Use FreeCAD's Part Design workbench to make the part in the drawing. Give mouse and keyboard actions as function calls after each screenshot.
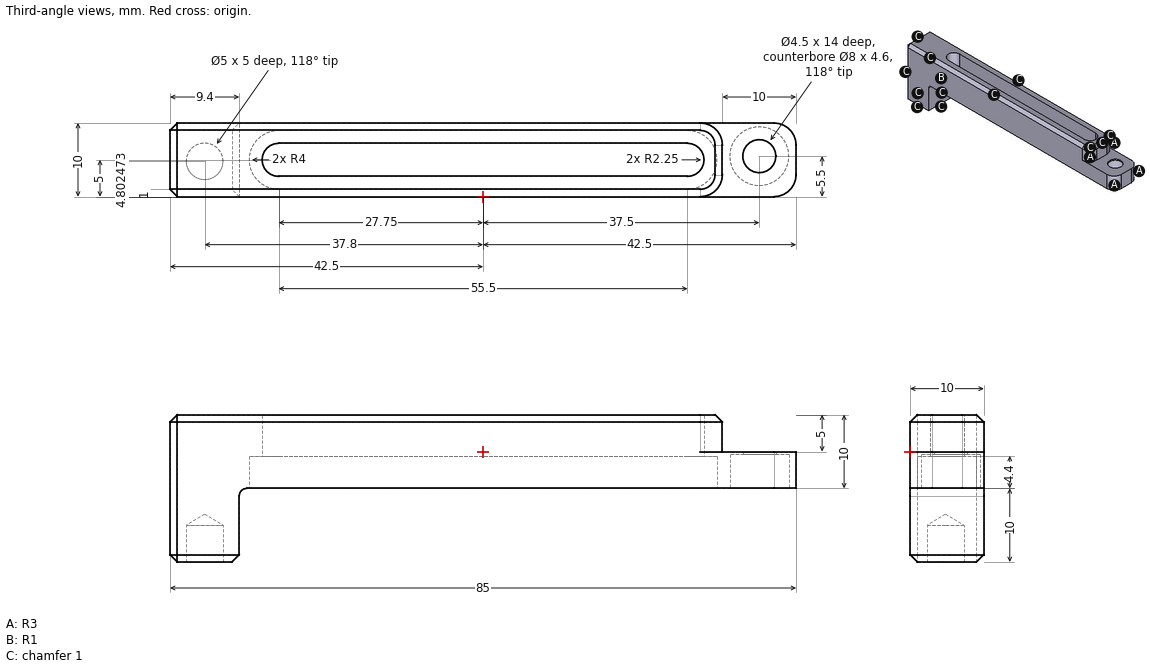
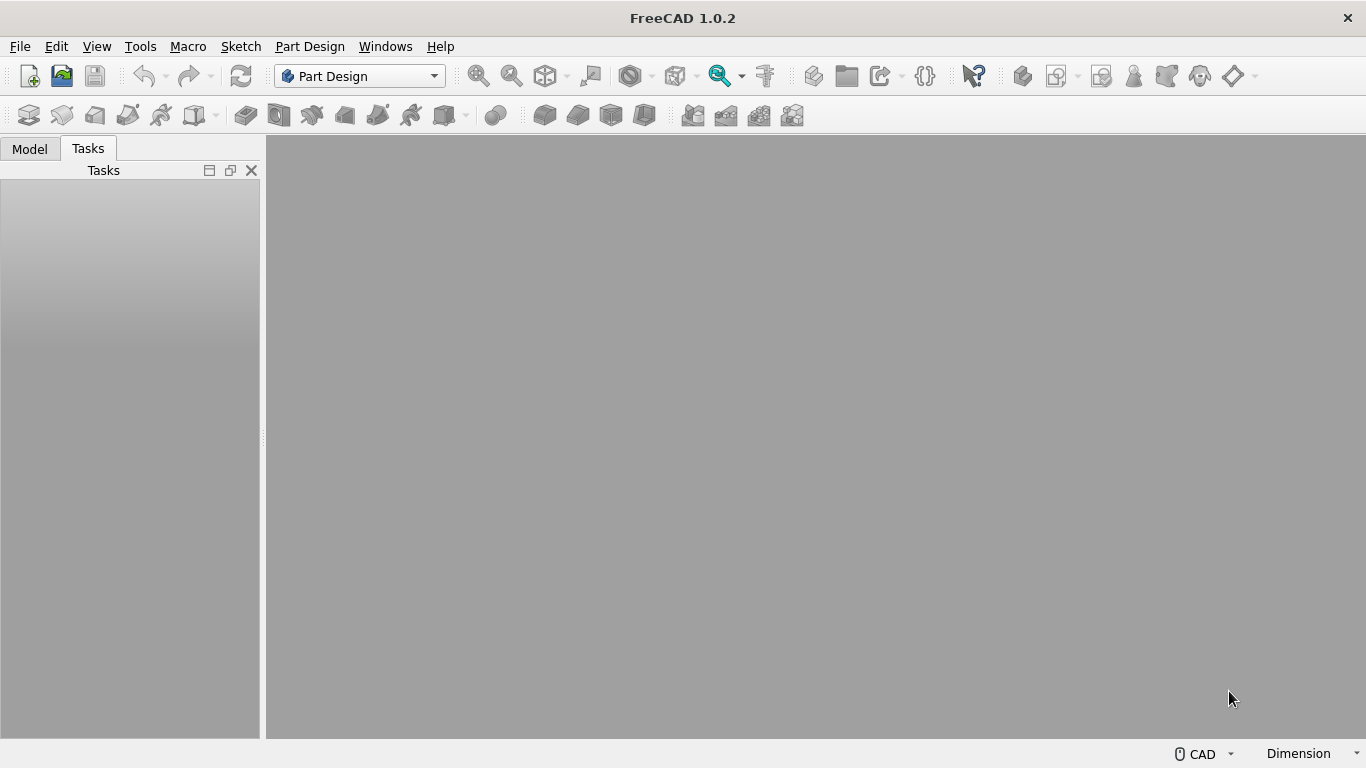
click(29, 76)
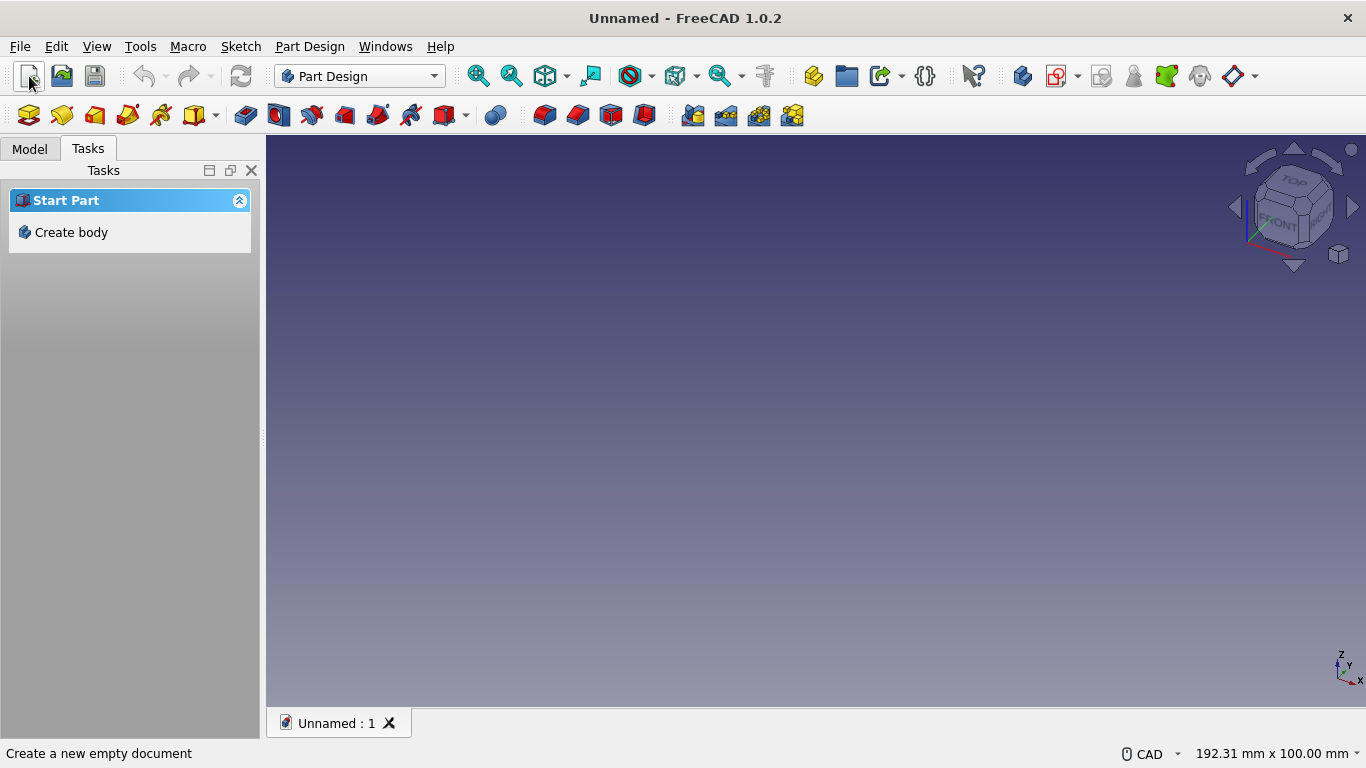
click(1056, 76)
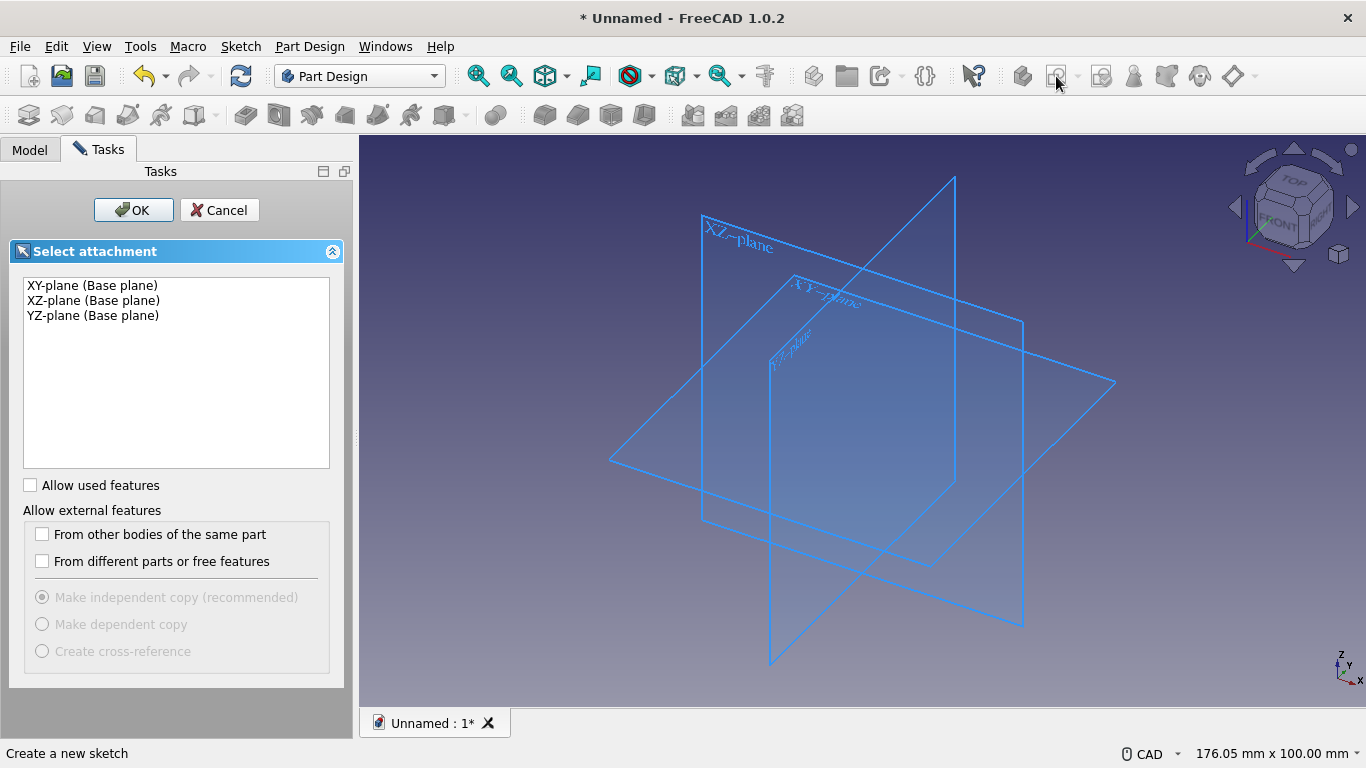
click(84, 300)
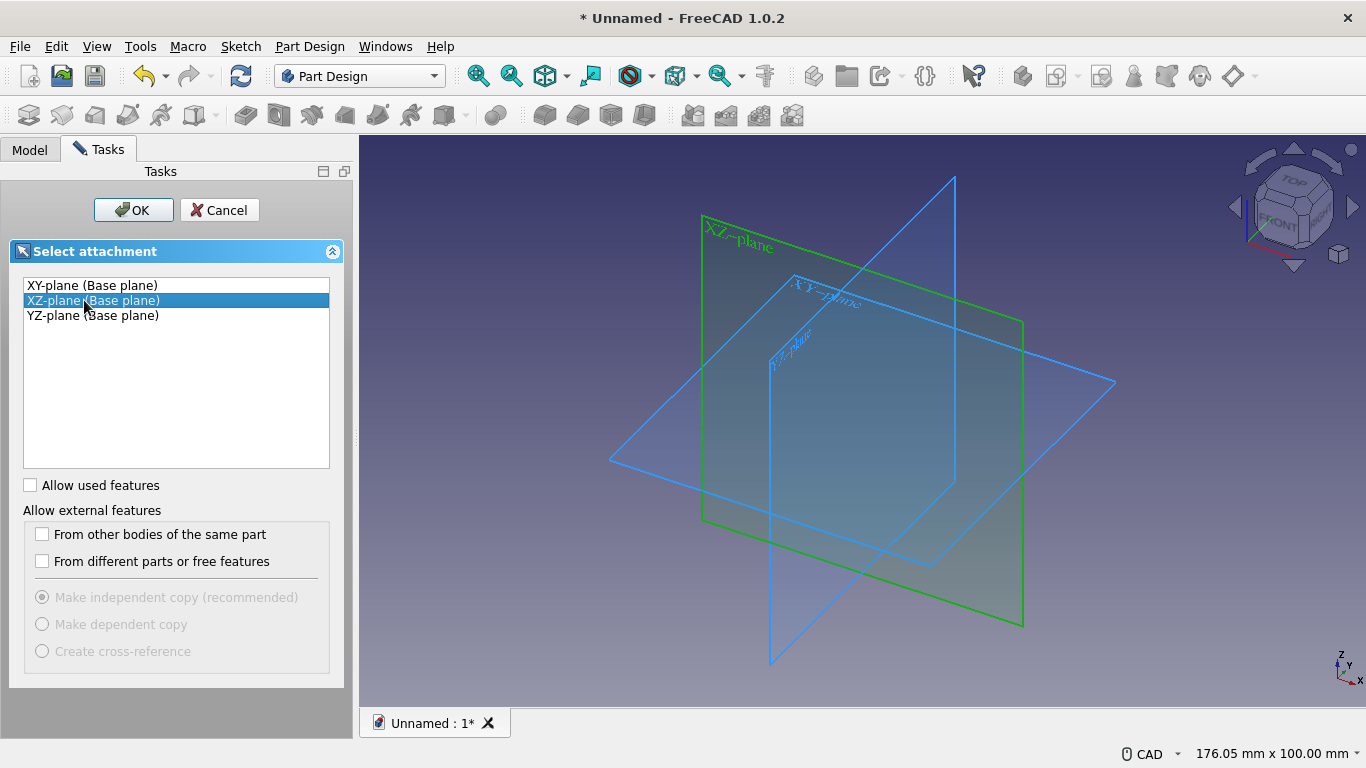
click(134, 210)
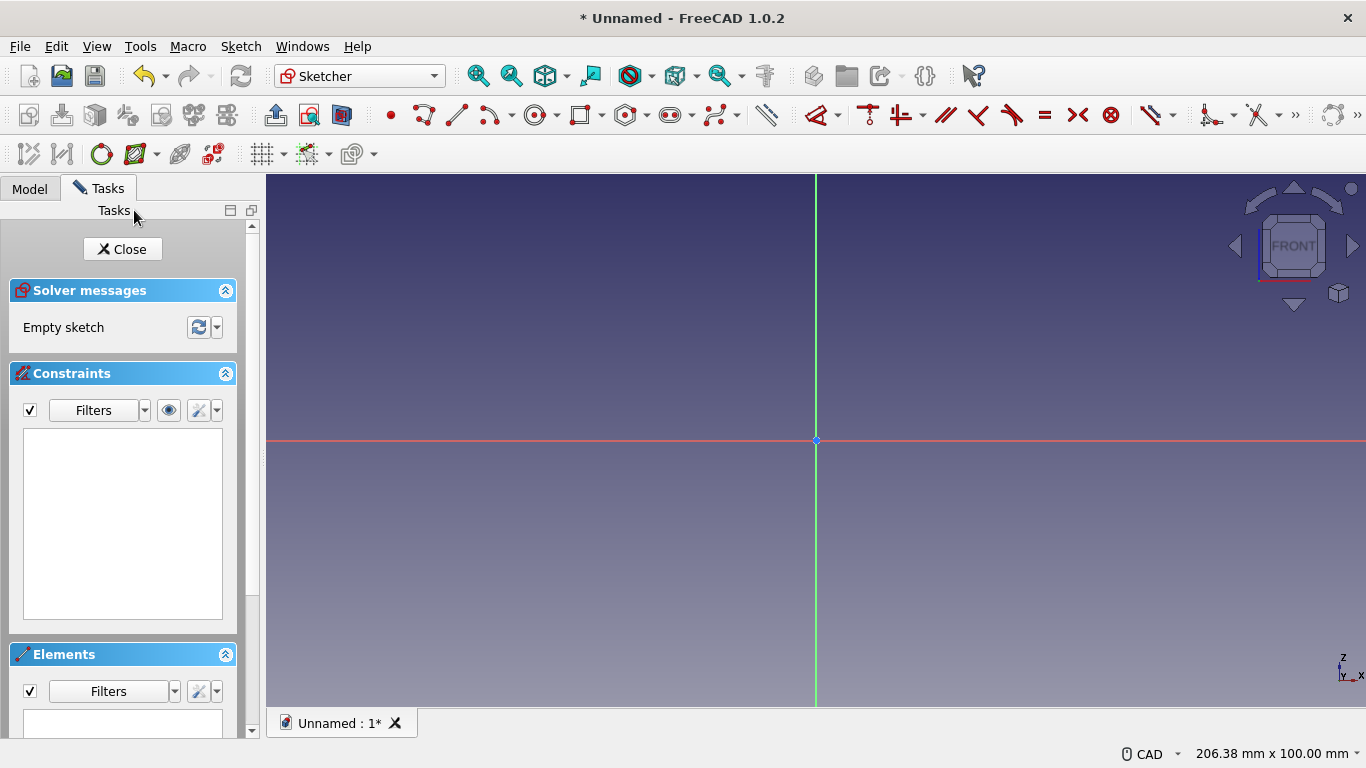
scroll(955, 440, up, 2)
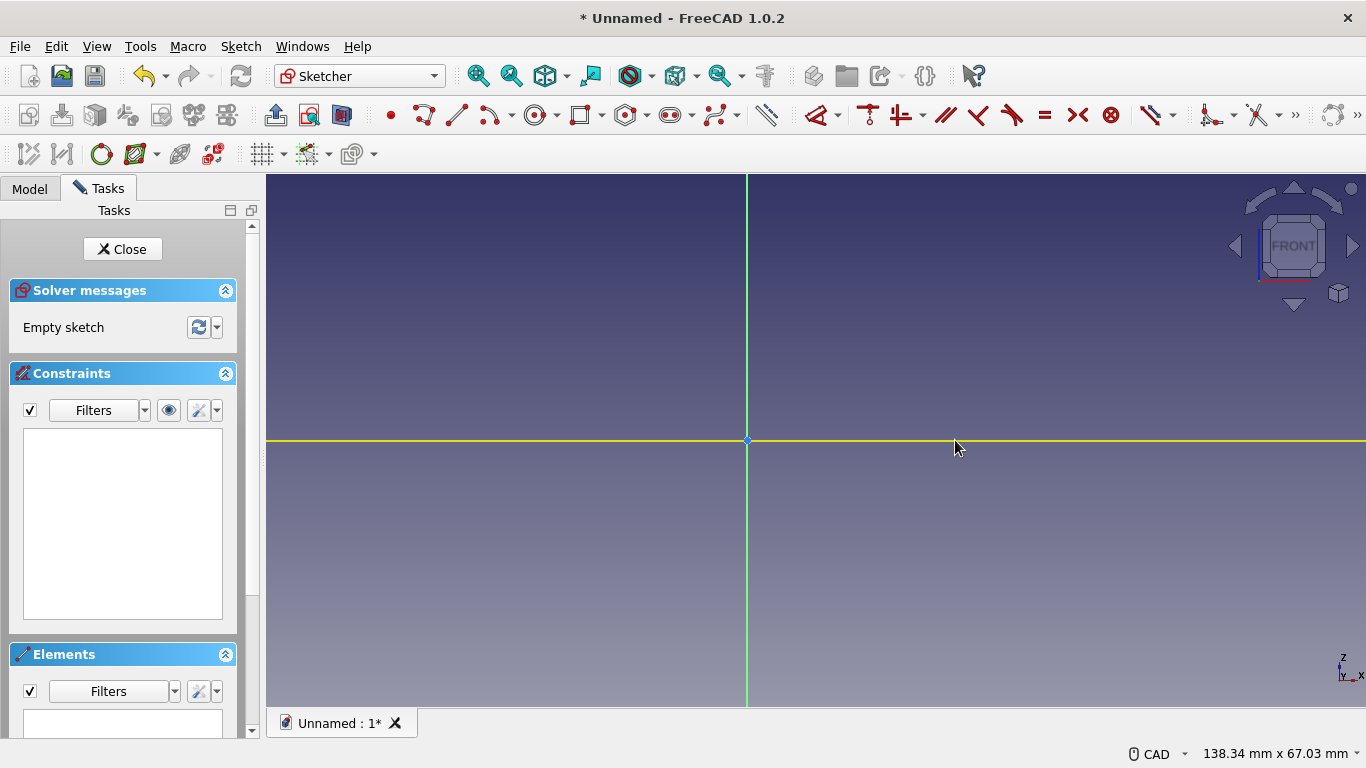
key(g)
key(v)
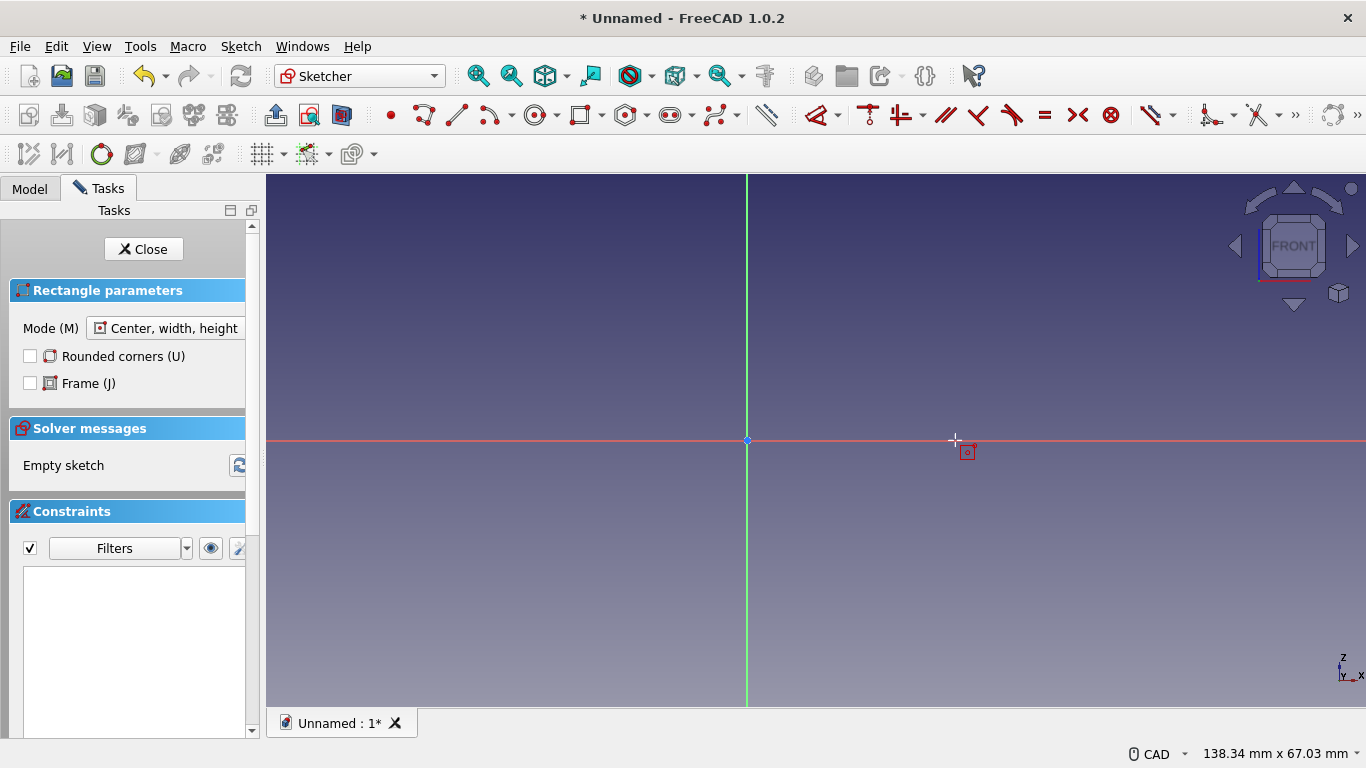
click(747, 440)
click(1085, 401)
key(Escape)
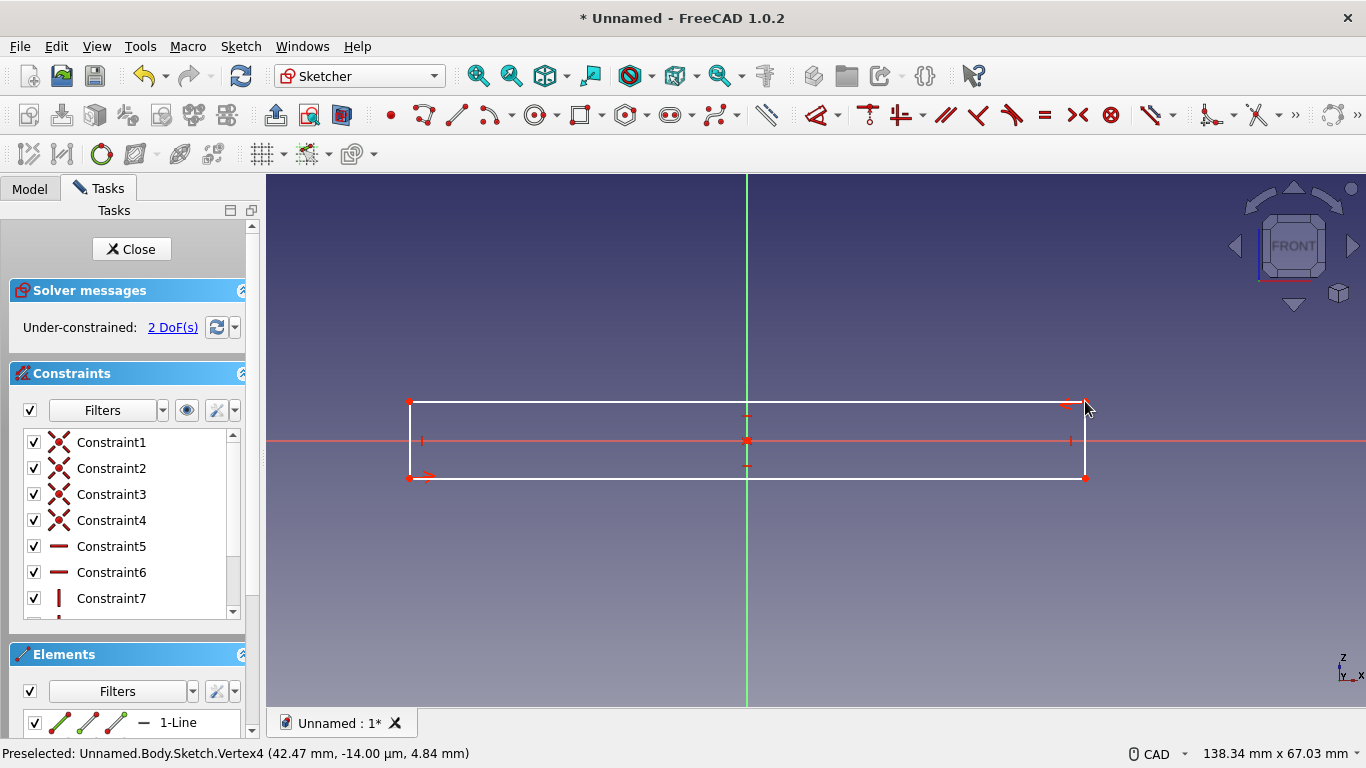
click(816, 116)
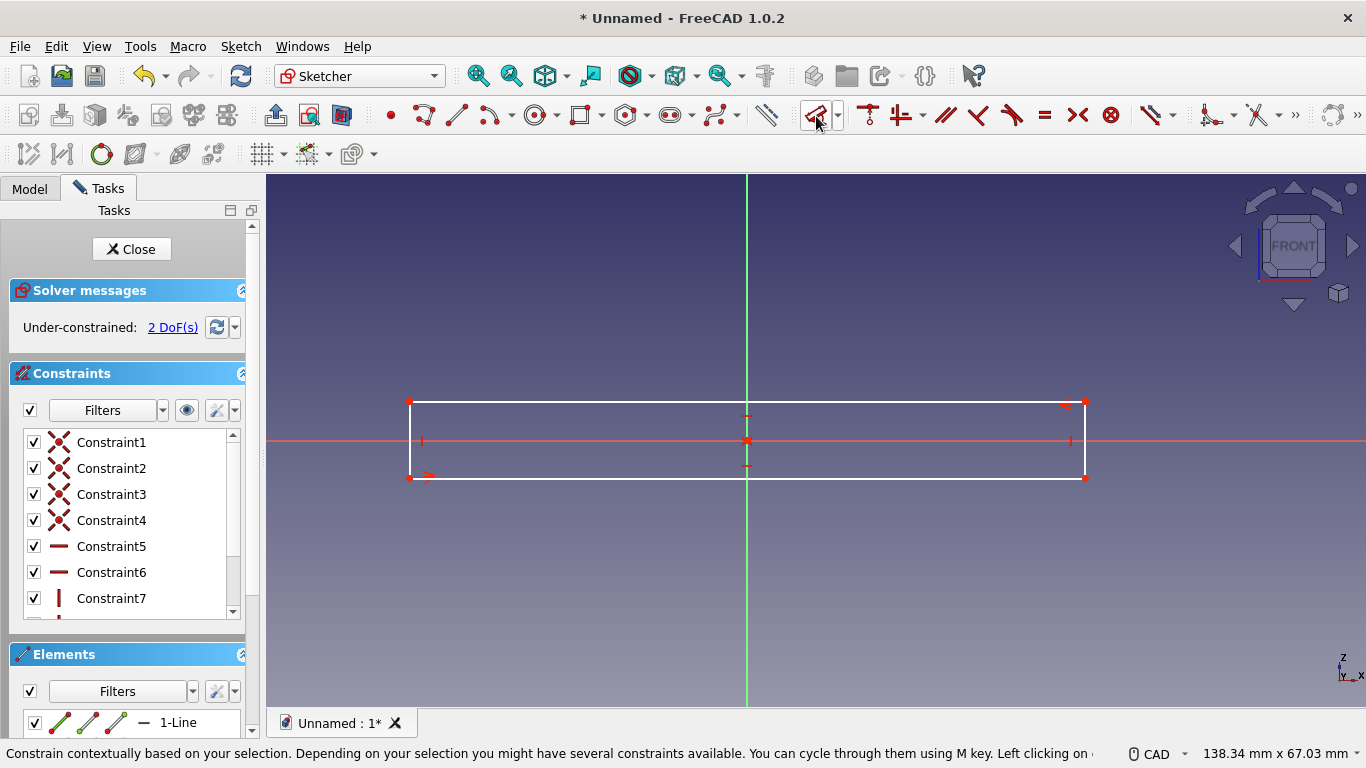
click(612, 479)
click(592, 513)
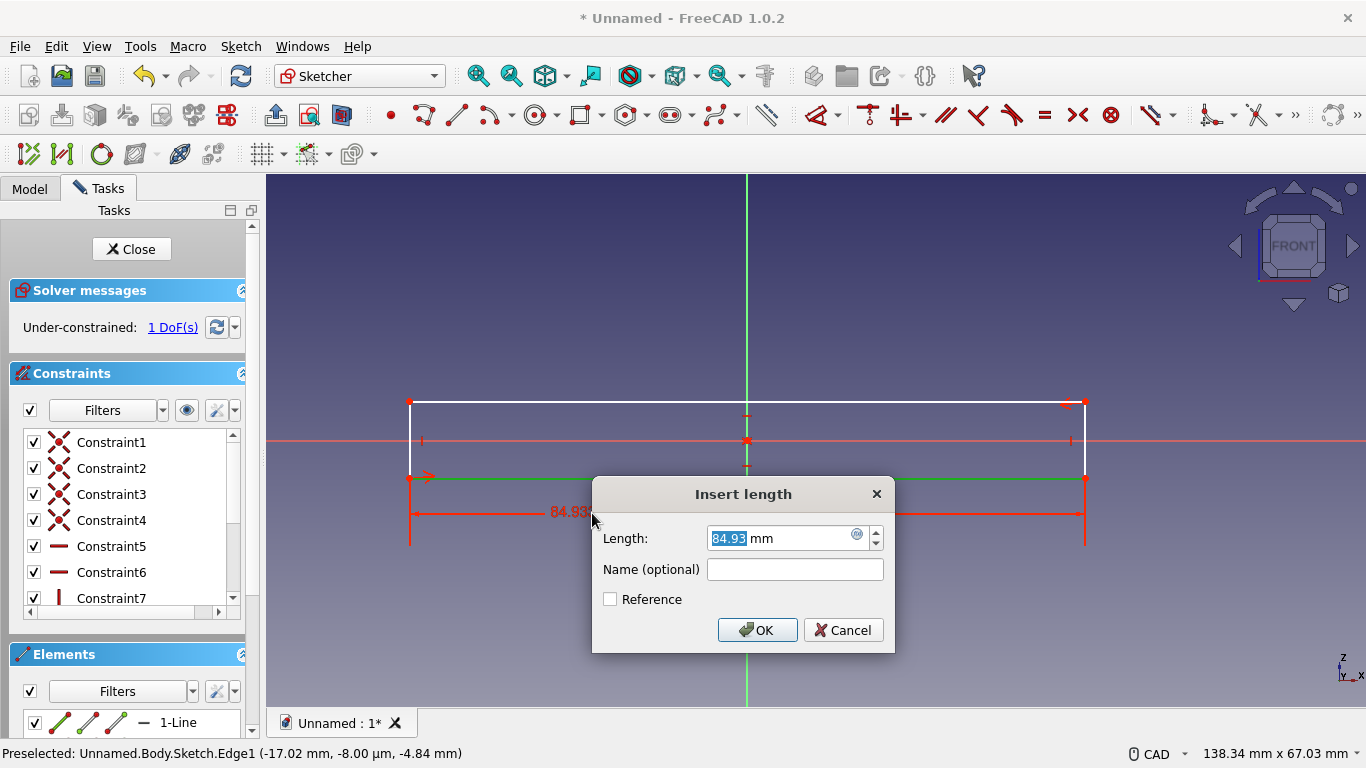
text(85)
key(Return)